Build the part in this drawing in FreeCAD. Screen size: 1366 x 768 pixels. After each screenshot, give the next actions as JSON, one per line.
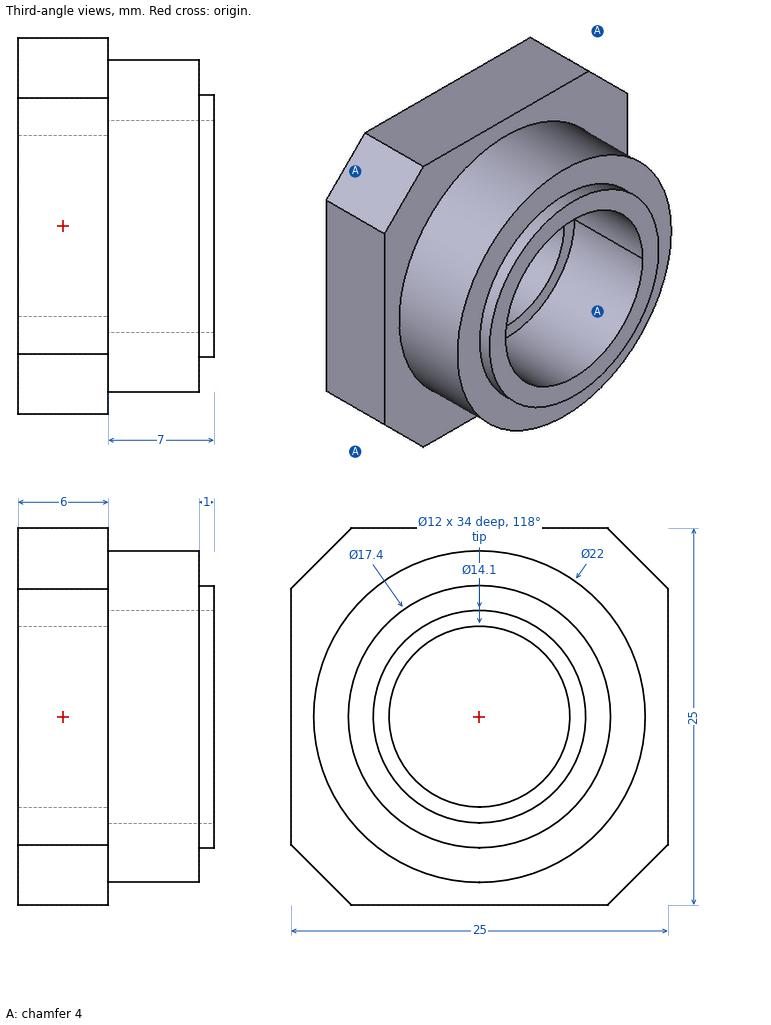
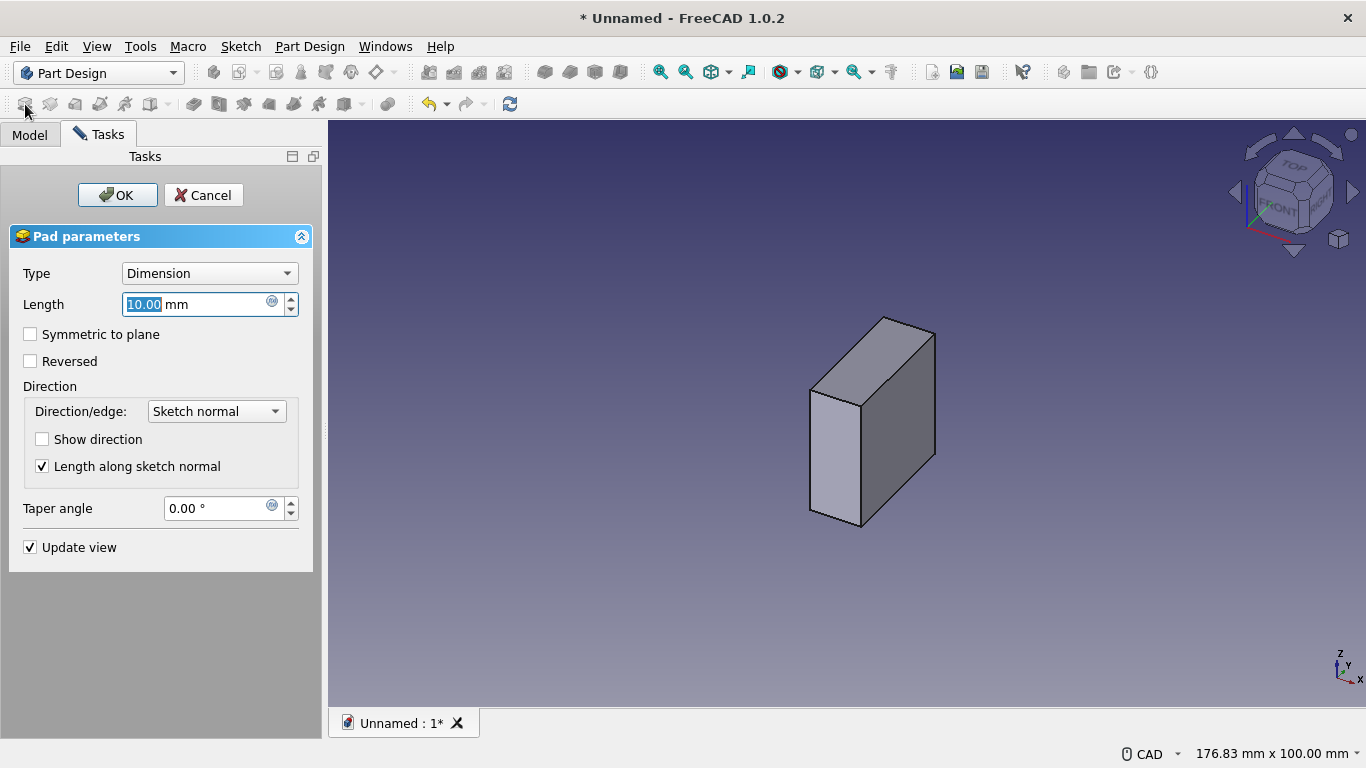
{"action": "type", "text": "6"}
{"action": "key", "text": "Tab"}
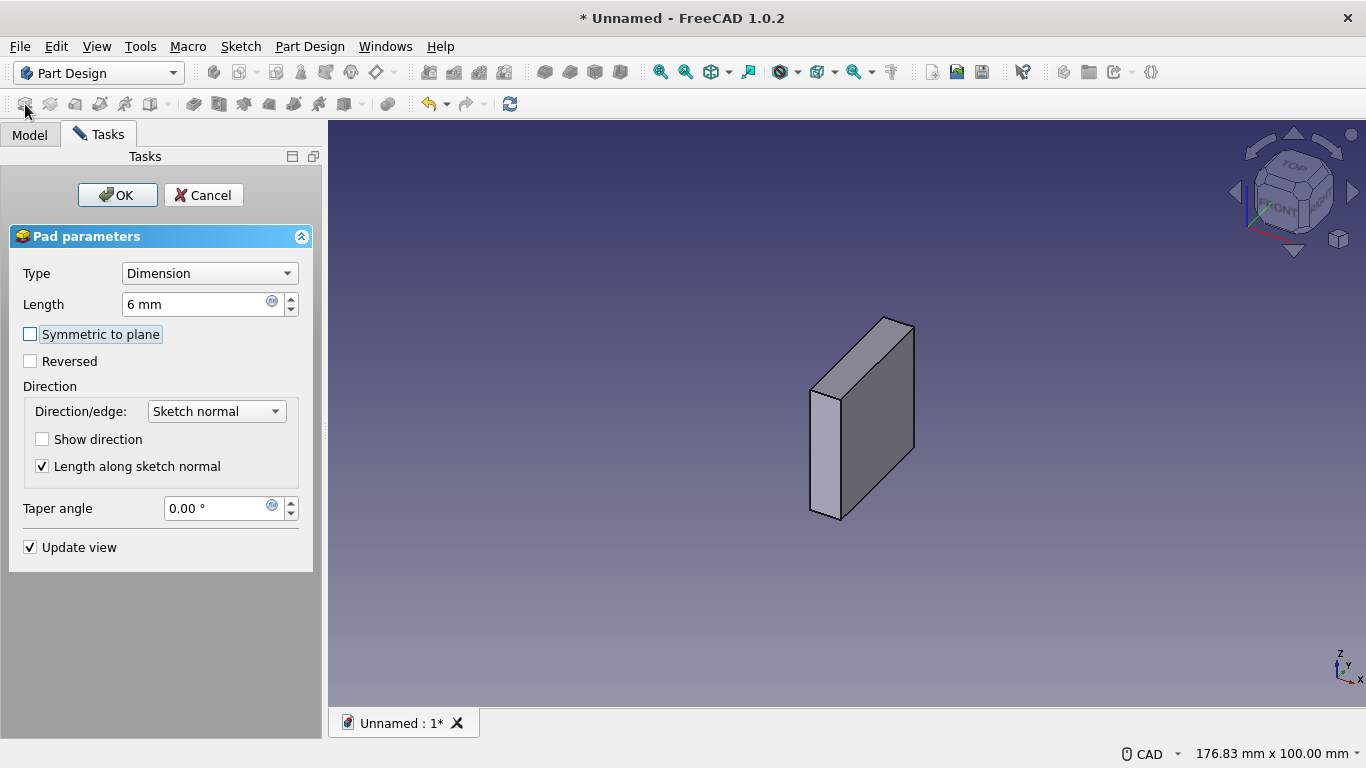
{"action": "left_click", "coordinate": [31, 334]}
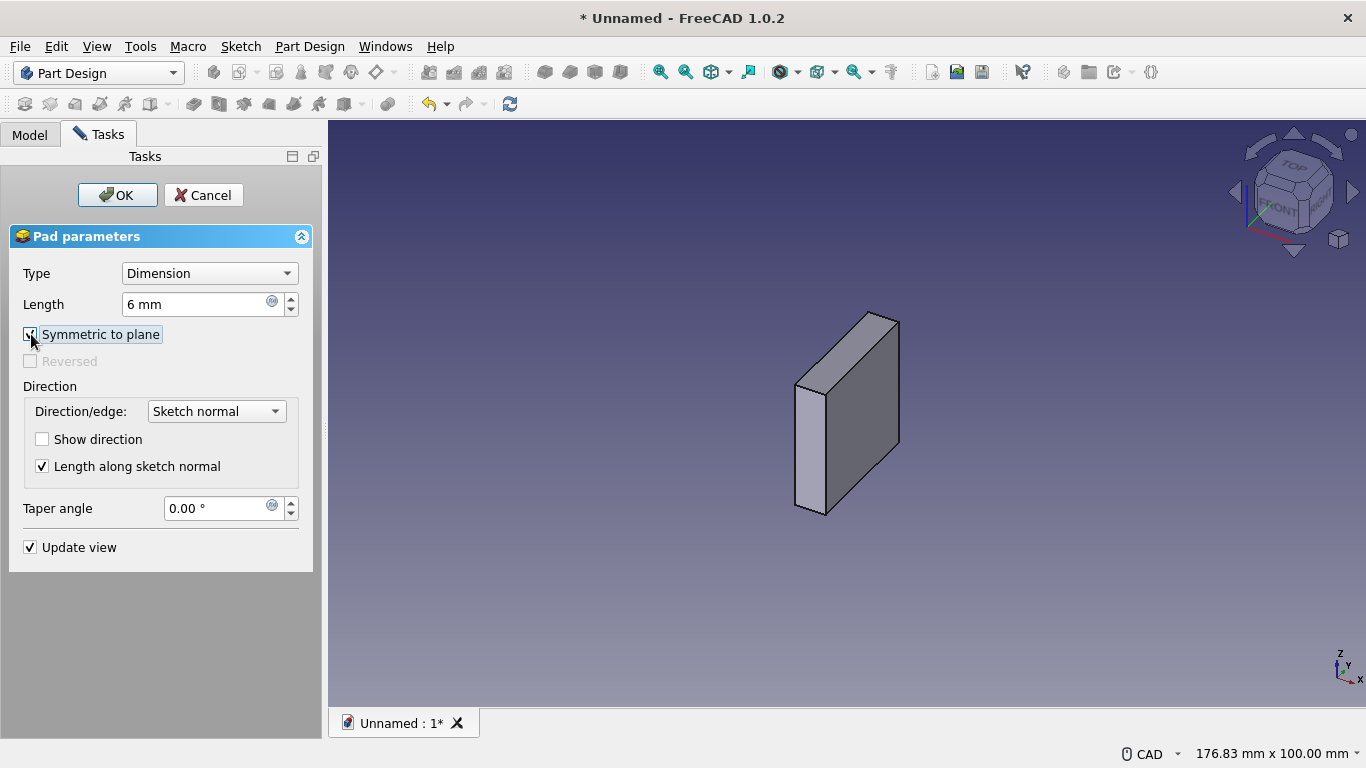
{"action": "left_click", "coordinate": [118, 195]}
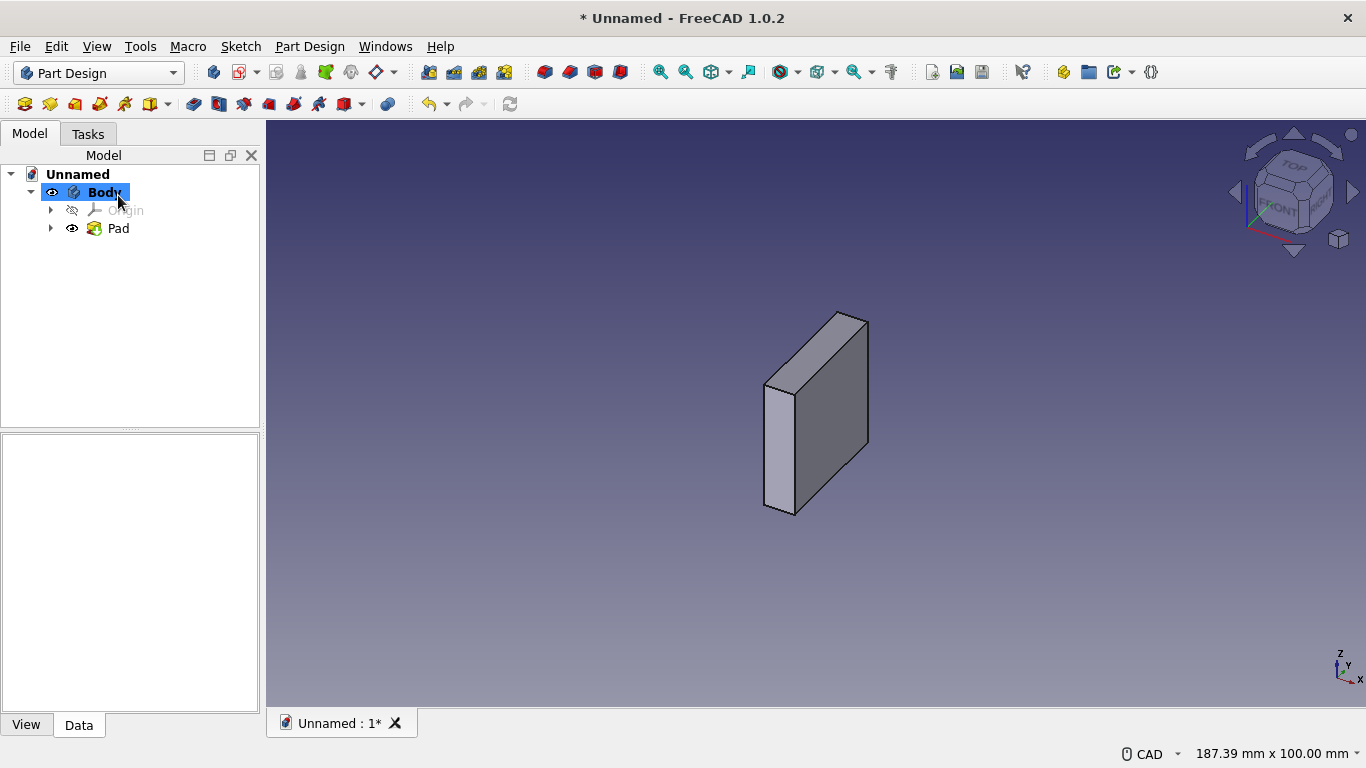
{"action": "left_click", "coordinate": [661, 72]}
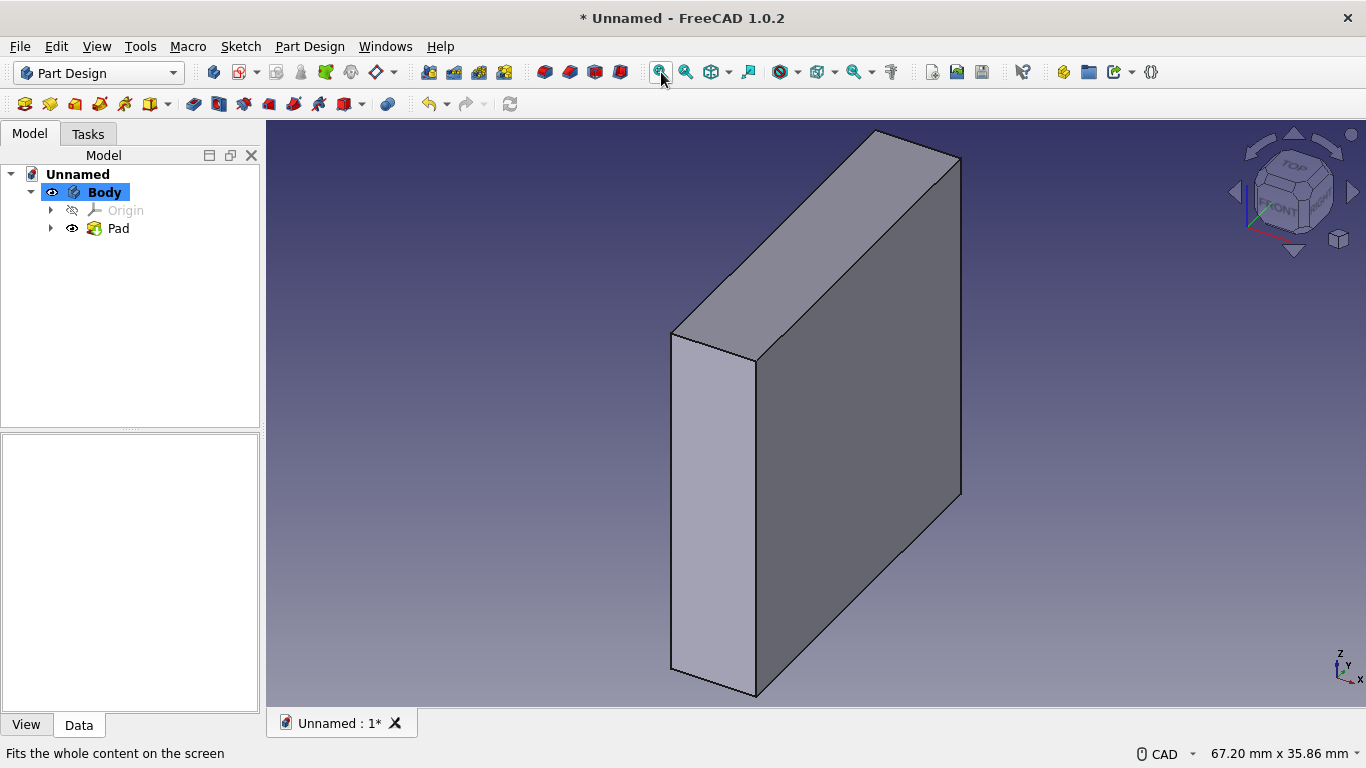
{"action": "key", "text": "6"}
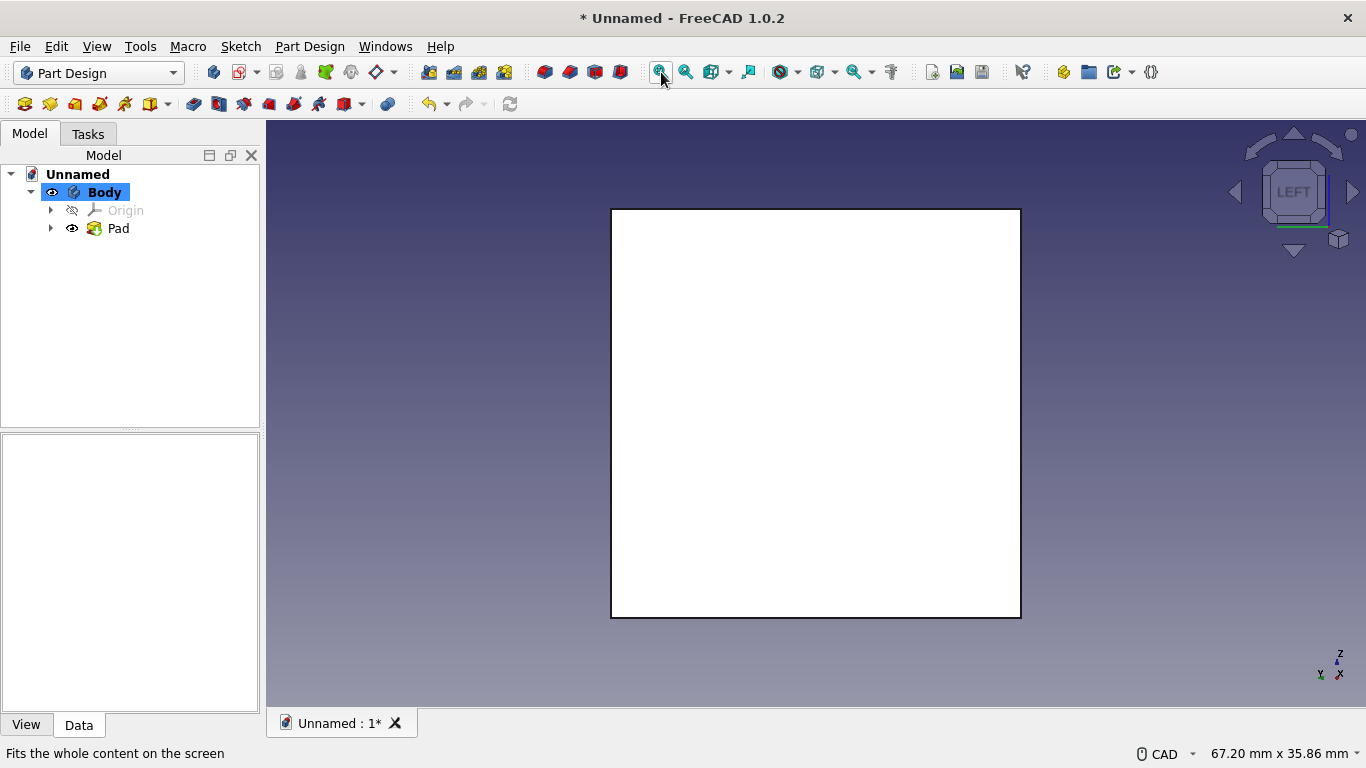
{"action": "left_click", "coordinate": [816, 412]}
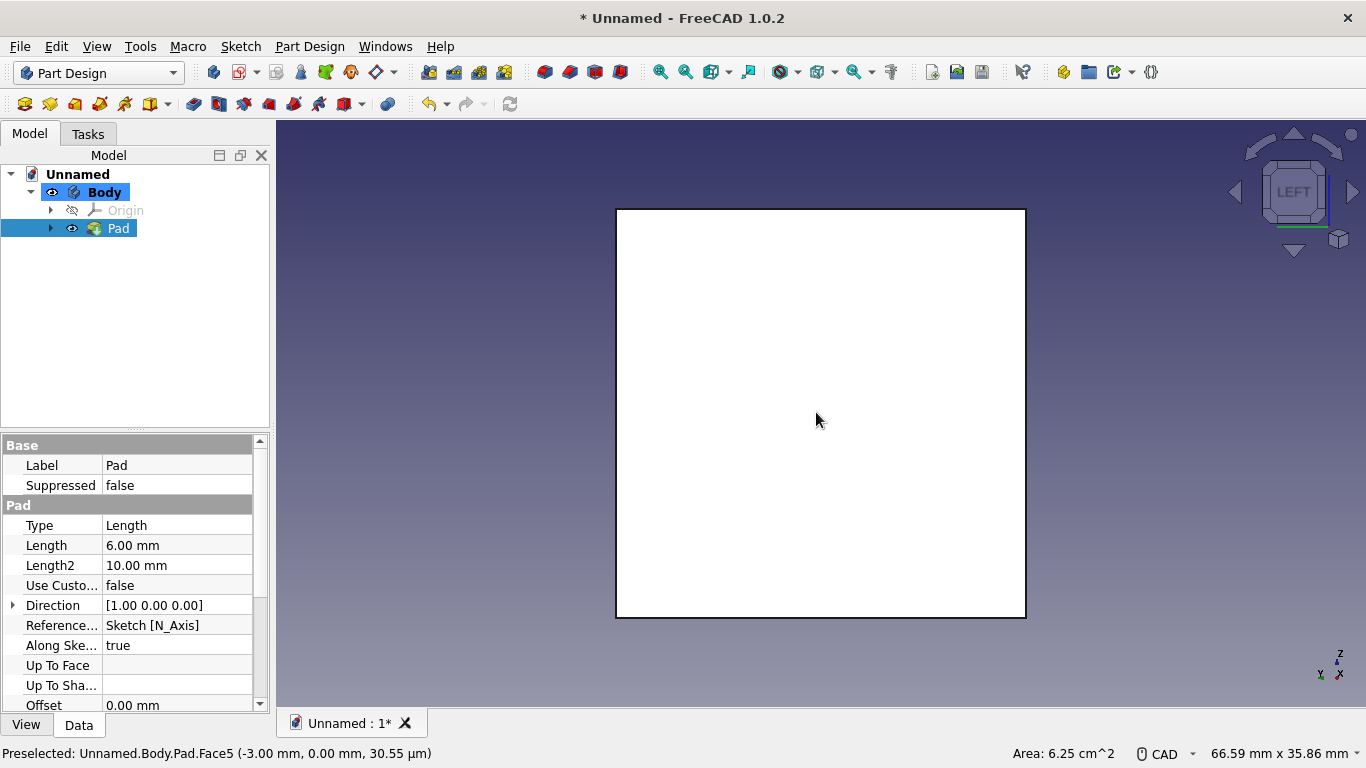
{"action": "left_click", "coordinate": [238, 72]}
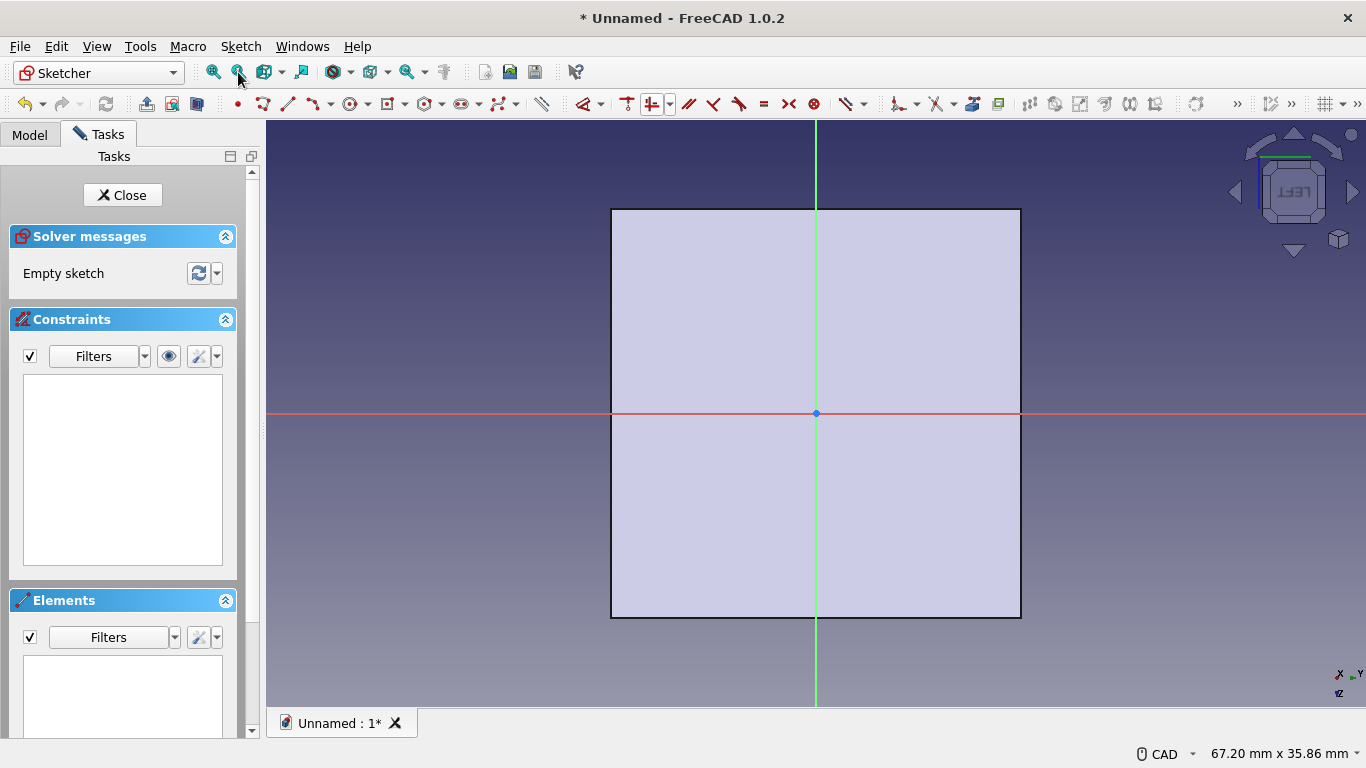
{"action": "scroll", "coordinate": [899, 414], "scroll_direction": "up", "scroll_amount": 3}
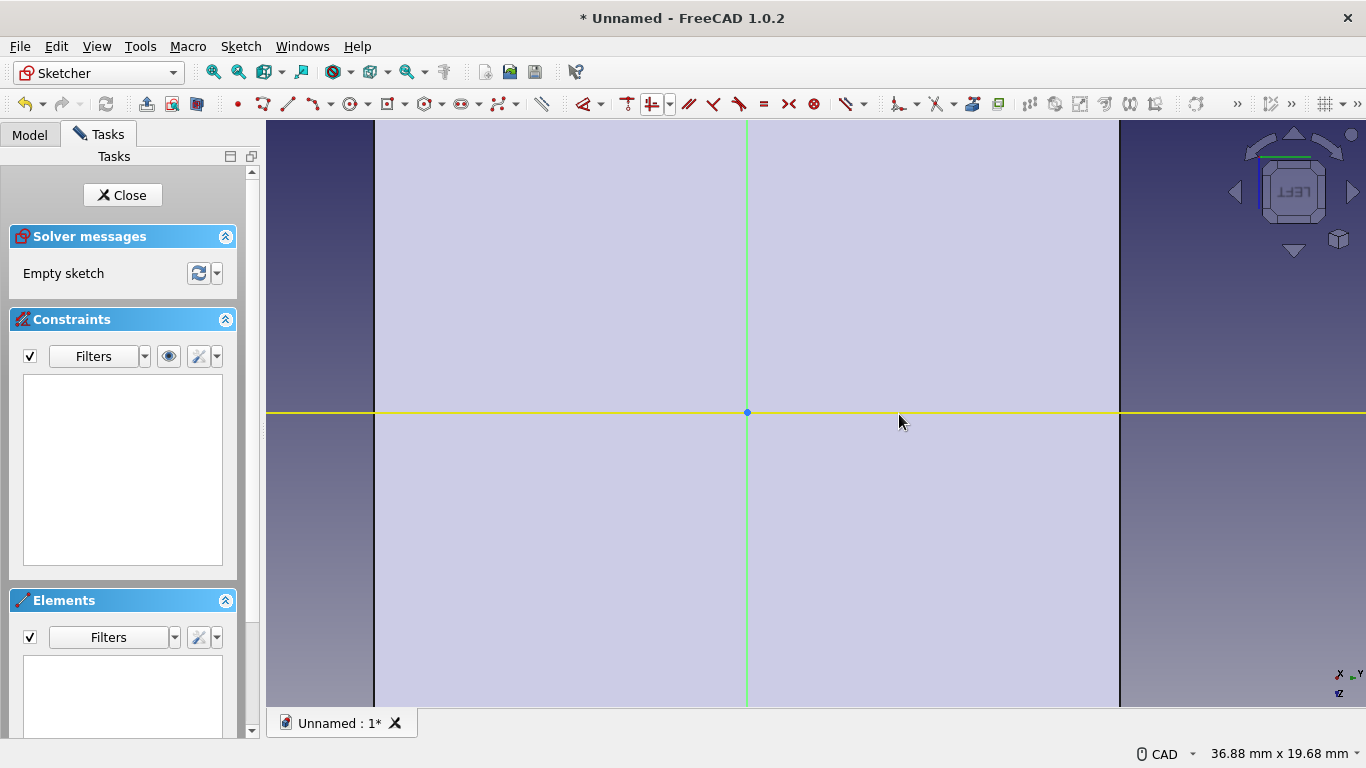
{"action": "left_click", "coordinate": [350, 104]}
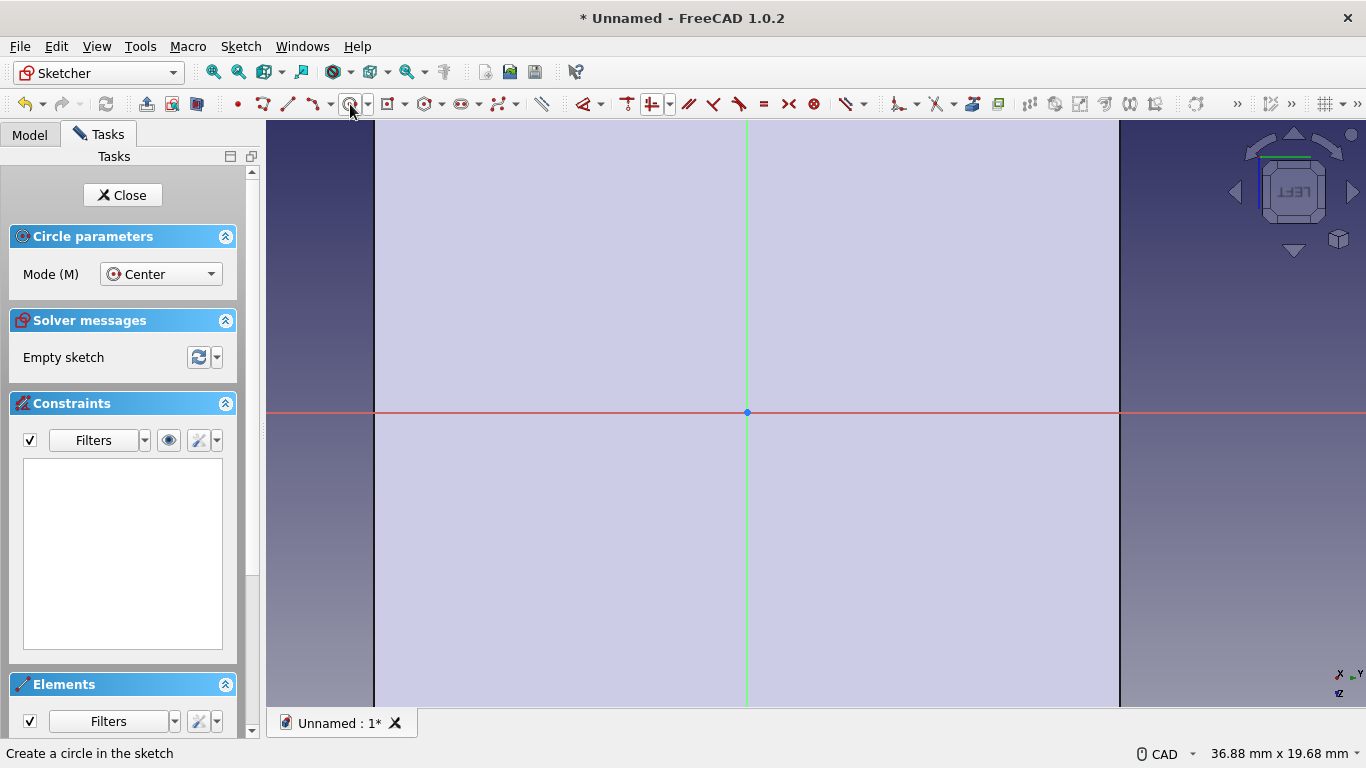
{"action": "left_click", "coordinate": [747, 413]}
{"action": "mouse_move", "coordinate": [874, 286]}